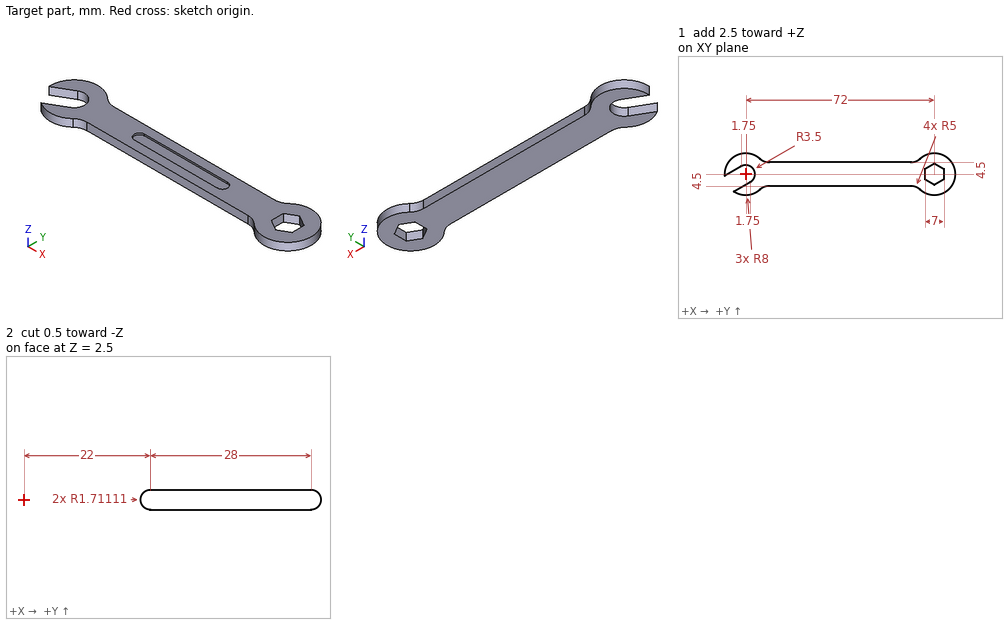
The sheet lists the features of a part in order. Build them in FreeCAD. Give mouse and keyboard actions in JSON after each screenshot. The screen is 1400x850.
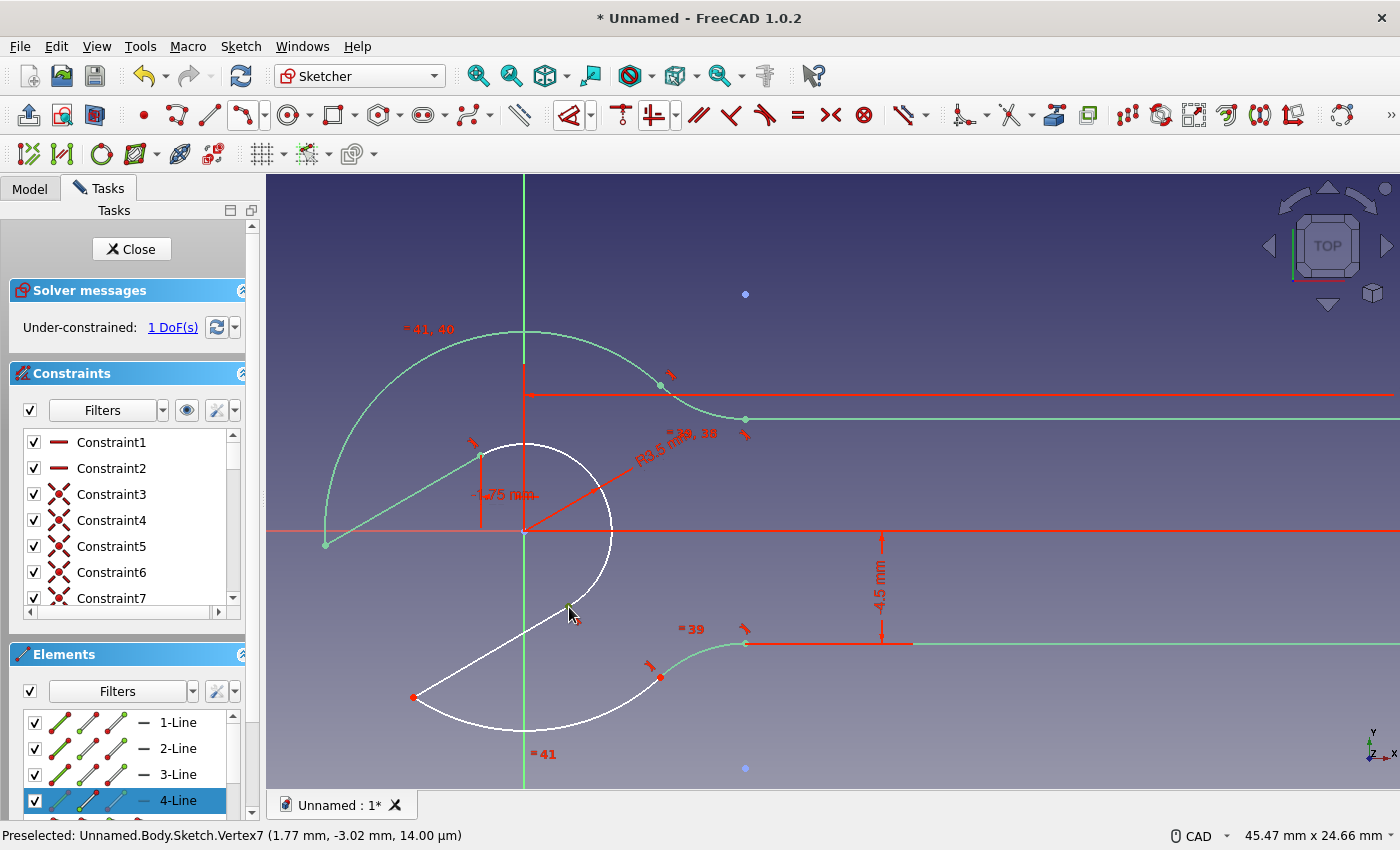
{"action": "left_click", "coordinate": [590, 116]}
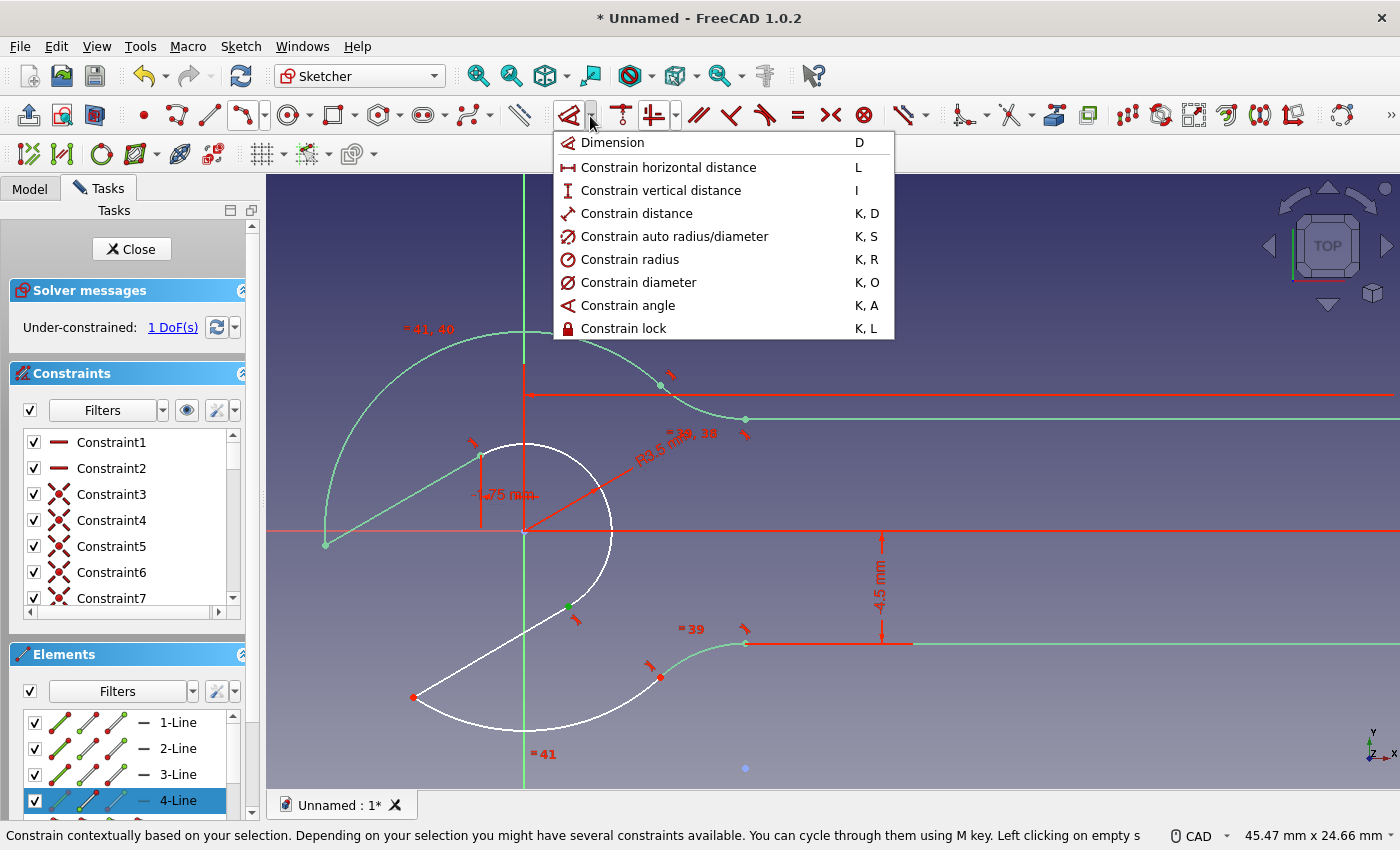
{"action": "left_click", "coordinate": [724, 168]}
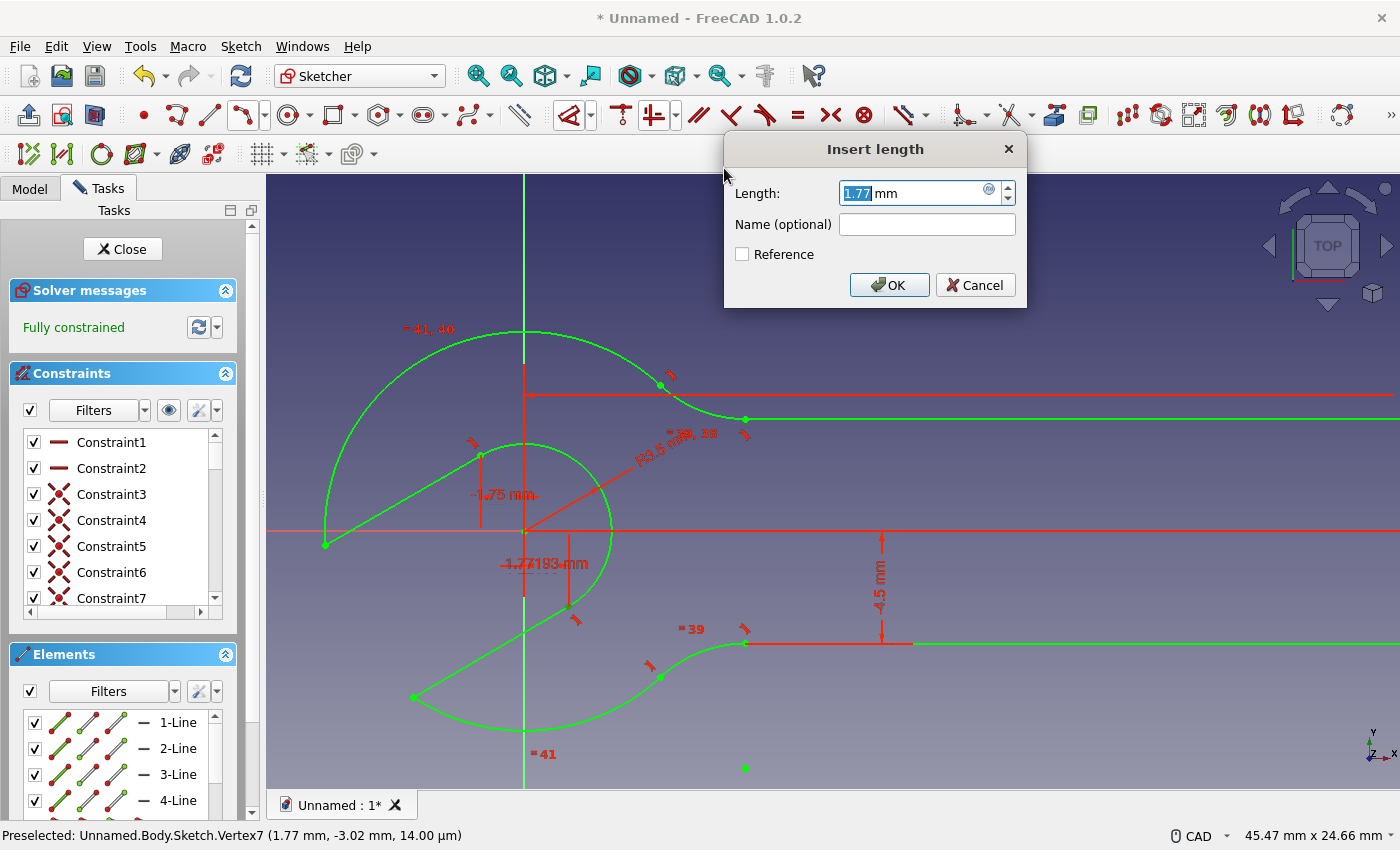
{"action": "type", "text": "1.75"}
{"action": "key", "text": "Return"}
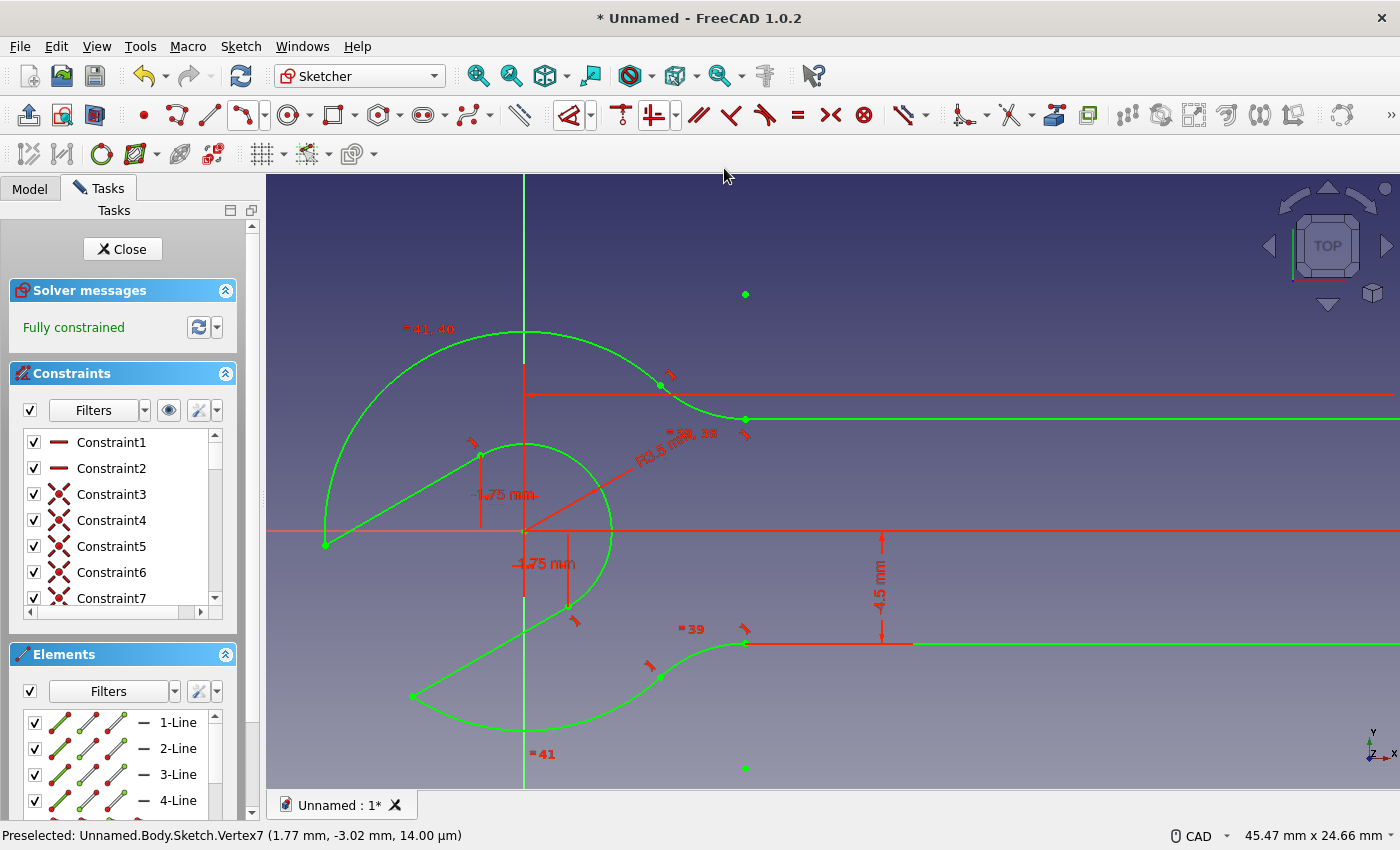
{"action": "left_click", "coordinate": [123, 249]}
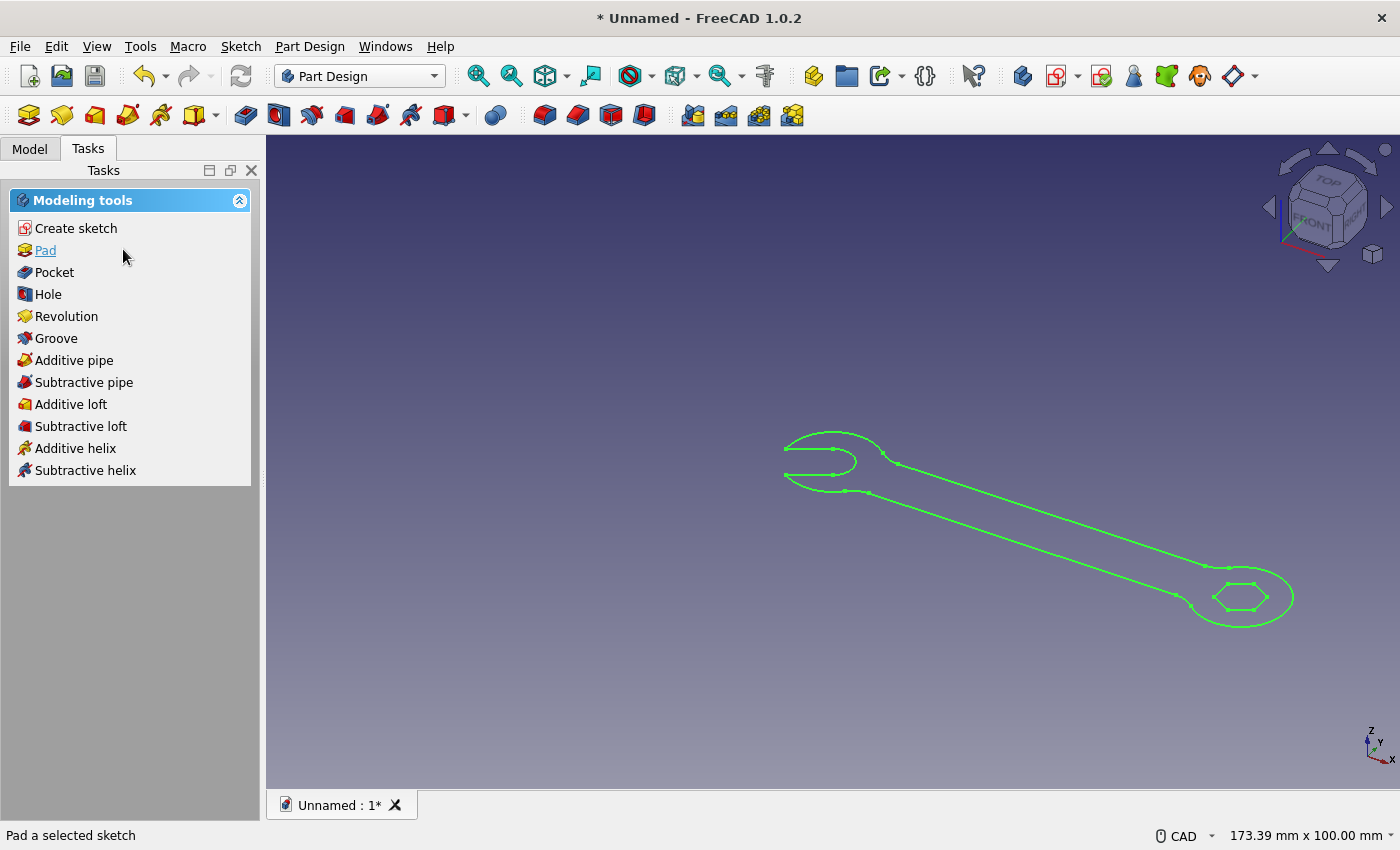
{"action": "left_click", "coordinate": [29, 116]}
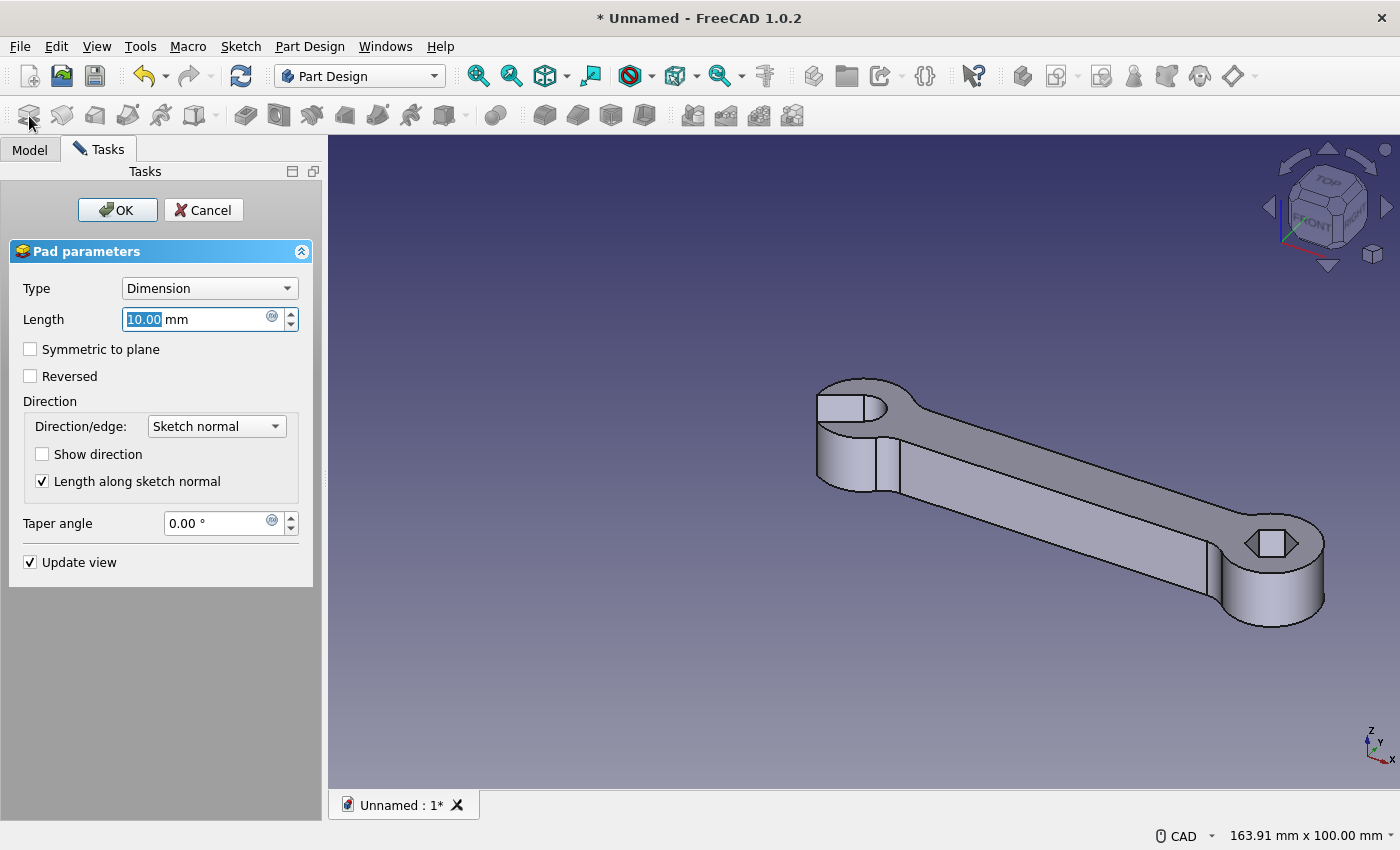
{"action": "type", "text": "2.5"}
{"action": "key", "text": "Tab"}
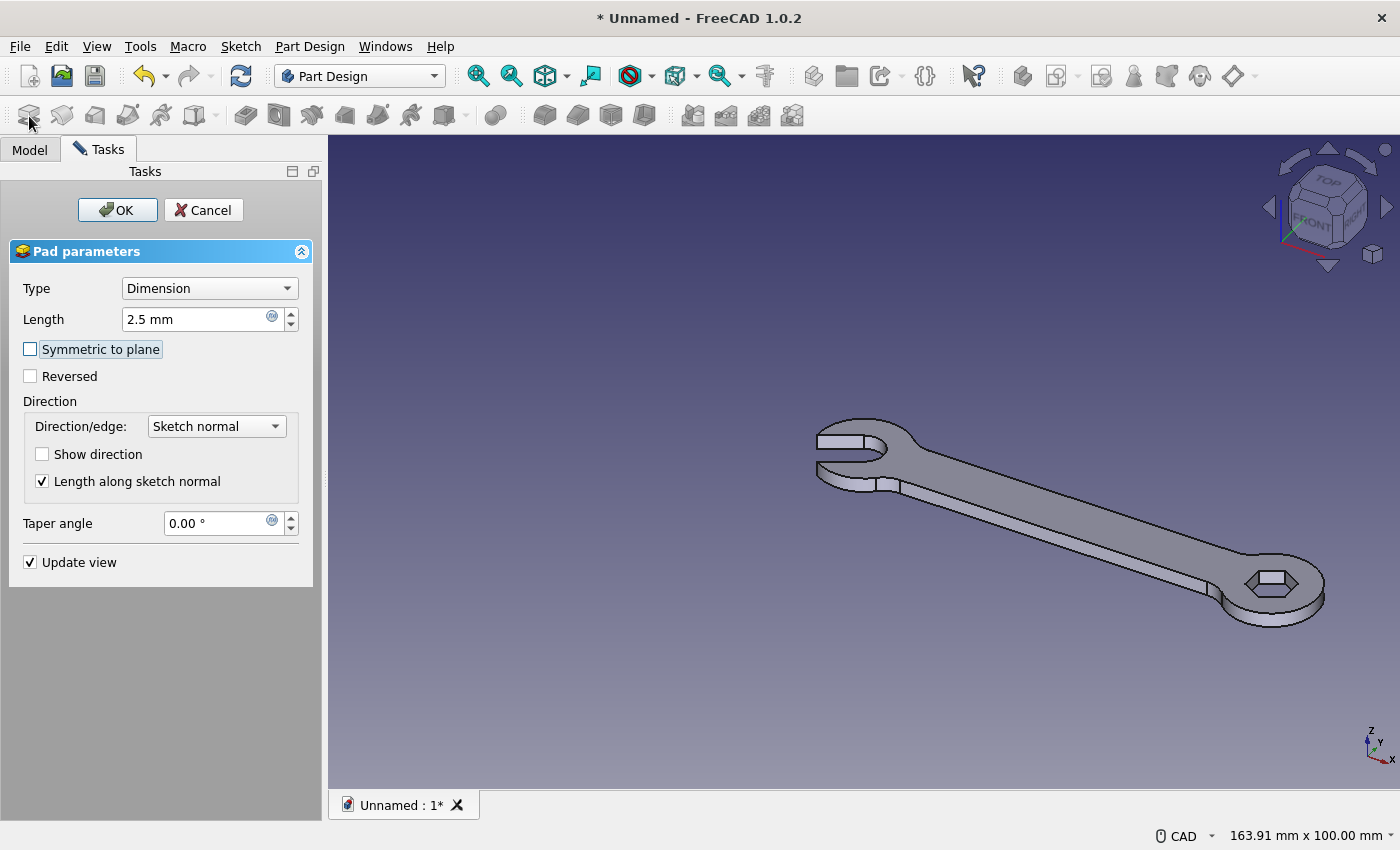
{"action": "left_click", "coordinate": [118, 210]}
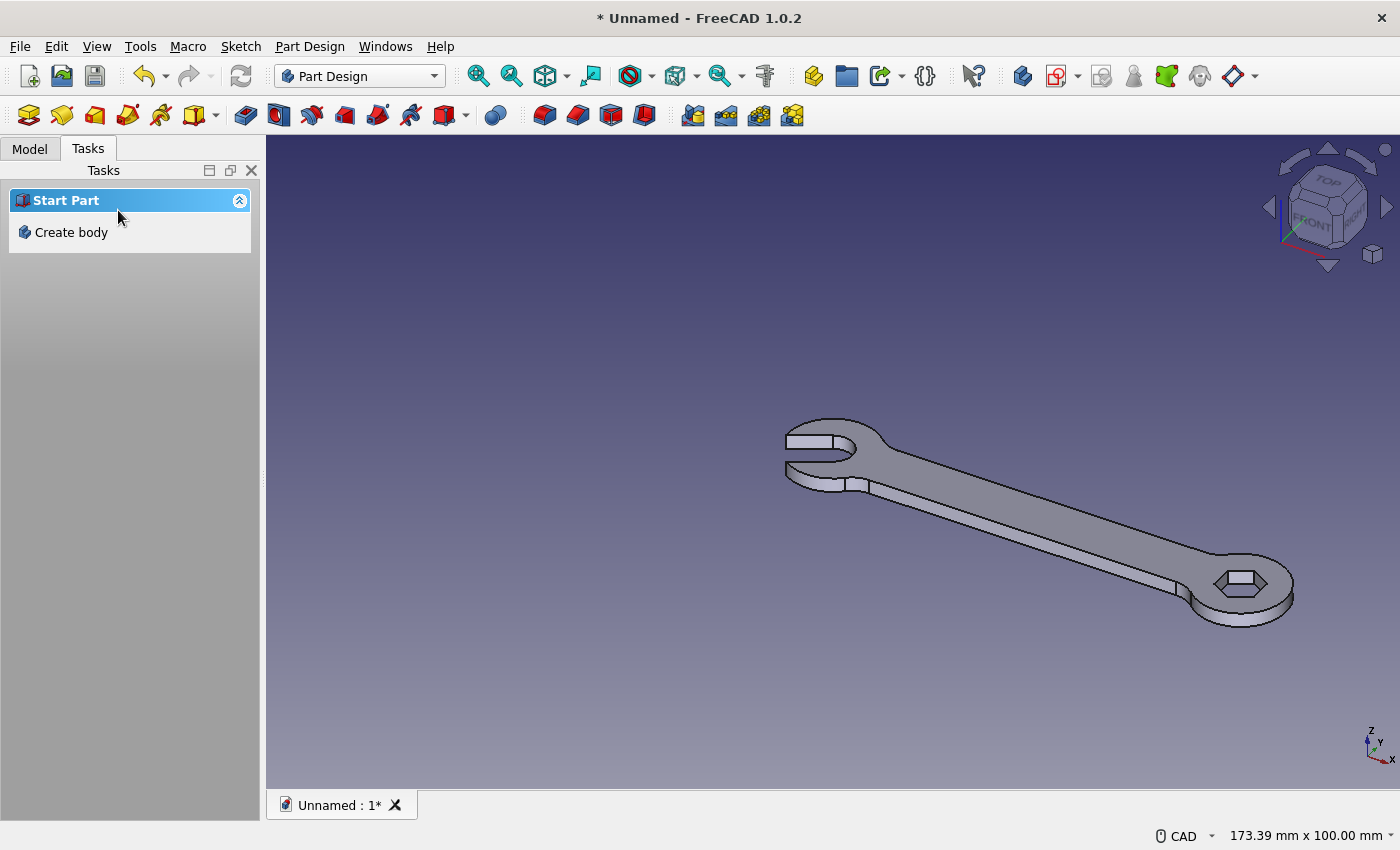
{"action": "left_click", "coordinate": [1179, 562]}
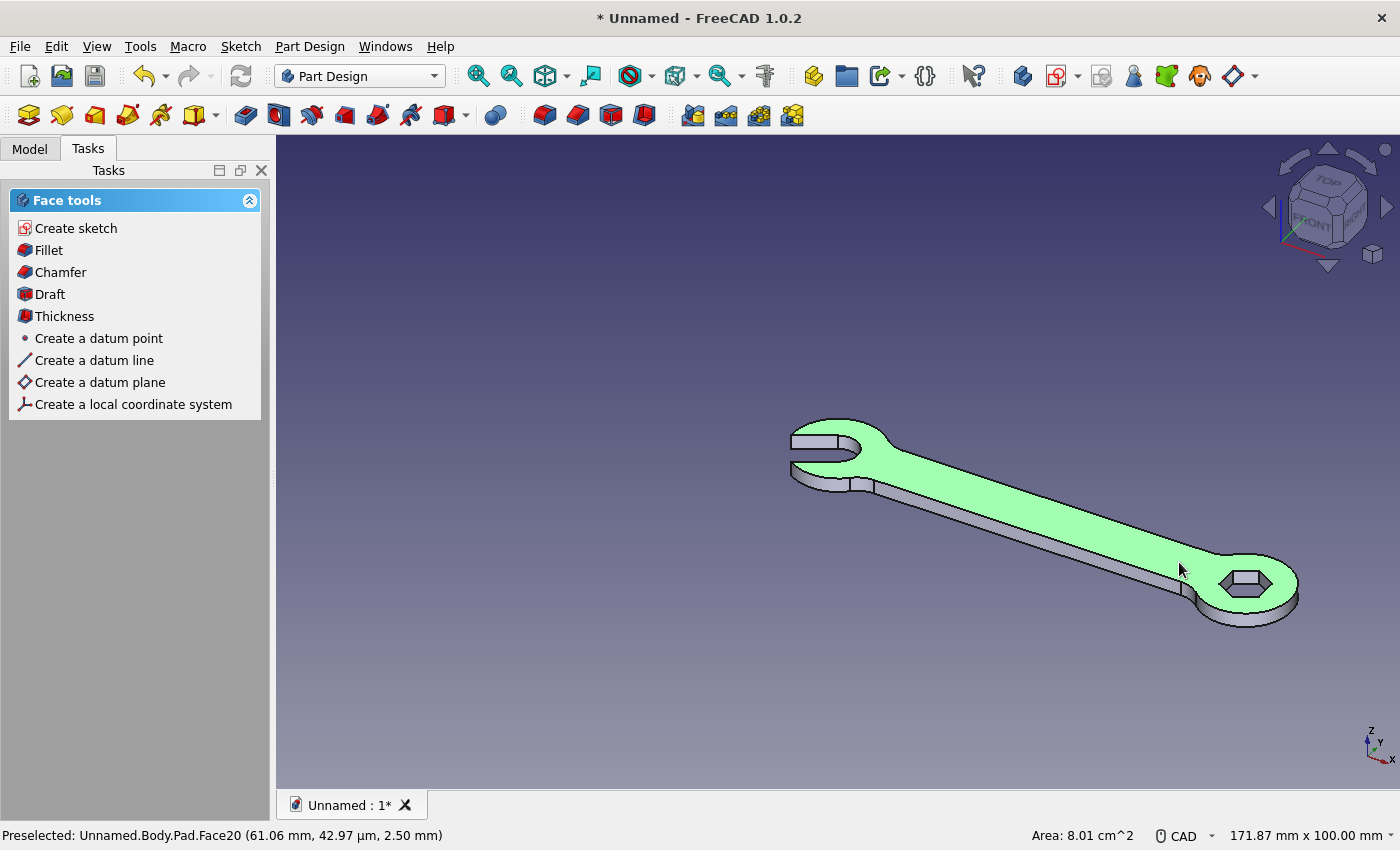
{"action": "left_click", "coordinate": [1056, 76]}